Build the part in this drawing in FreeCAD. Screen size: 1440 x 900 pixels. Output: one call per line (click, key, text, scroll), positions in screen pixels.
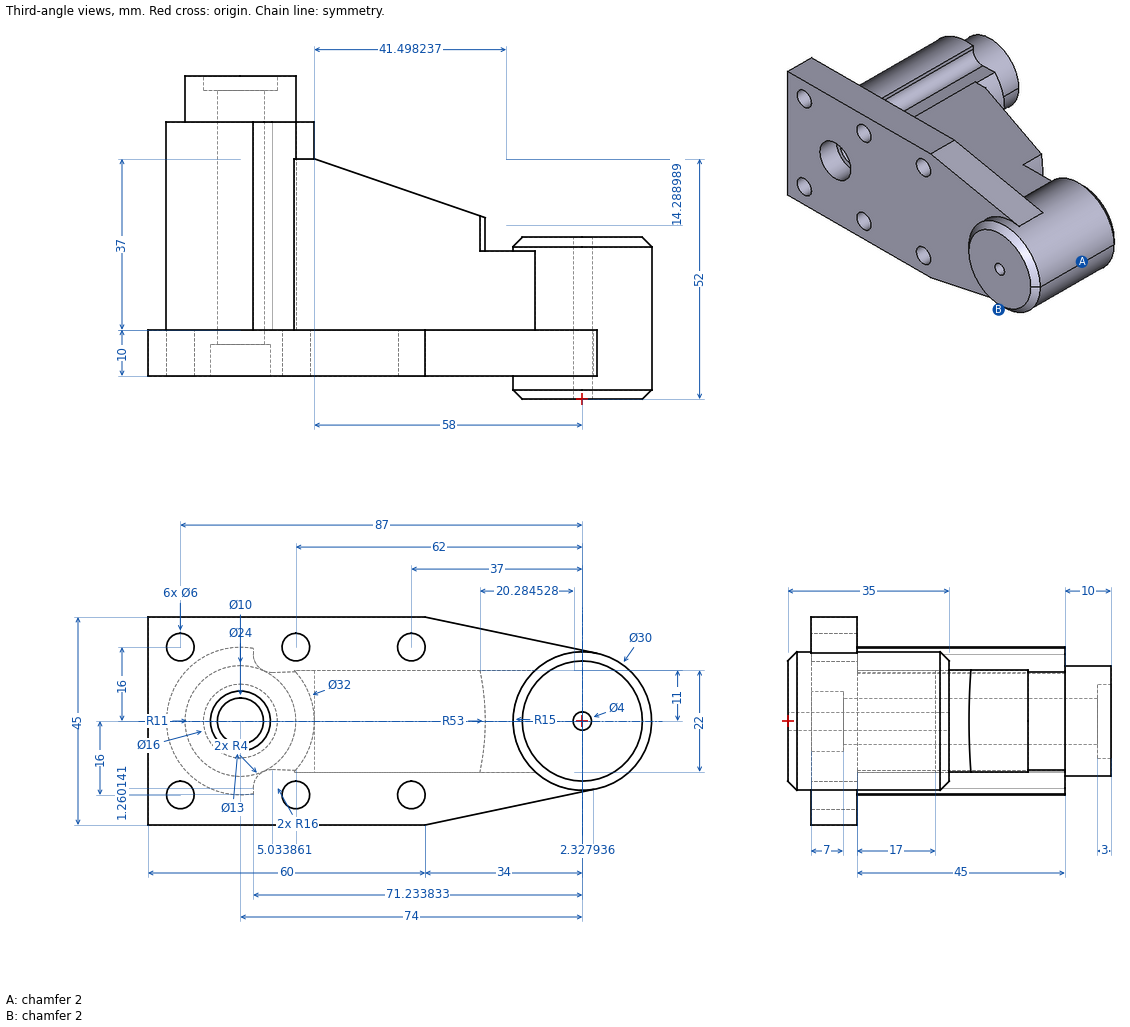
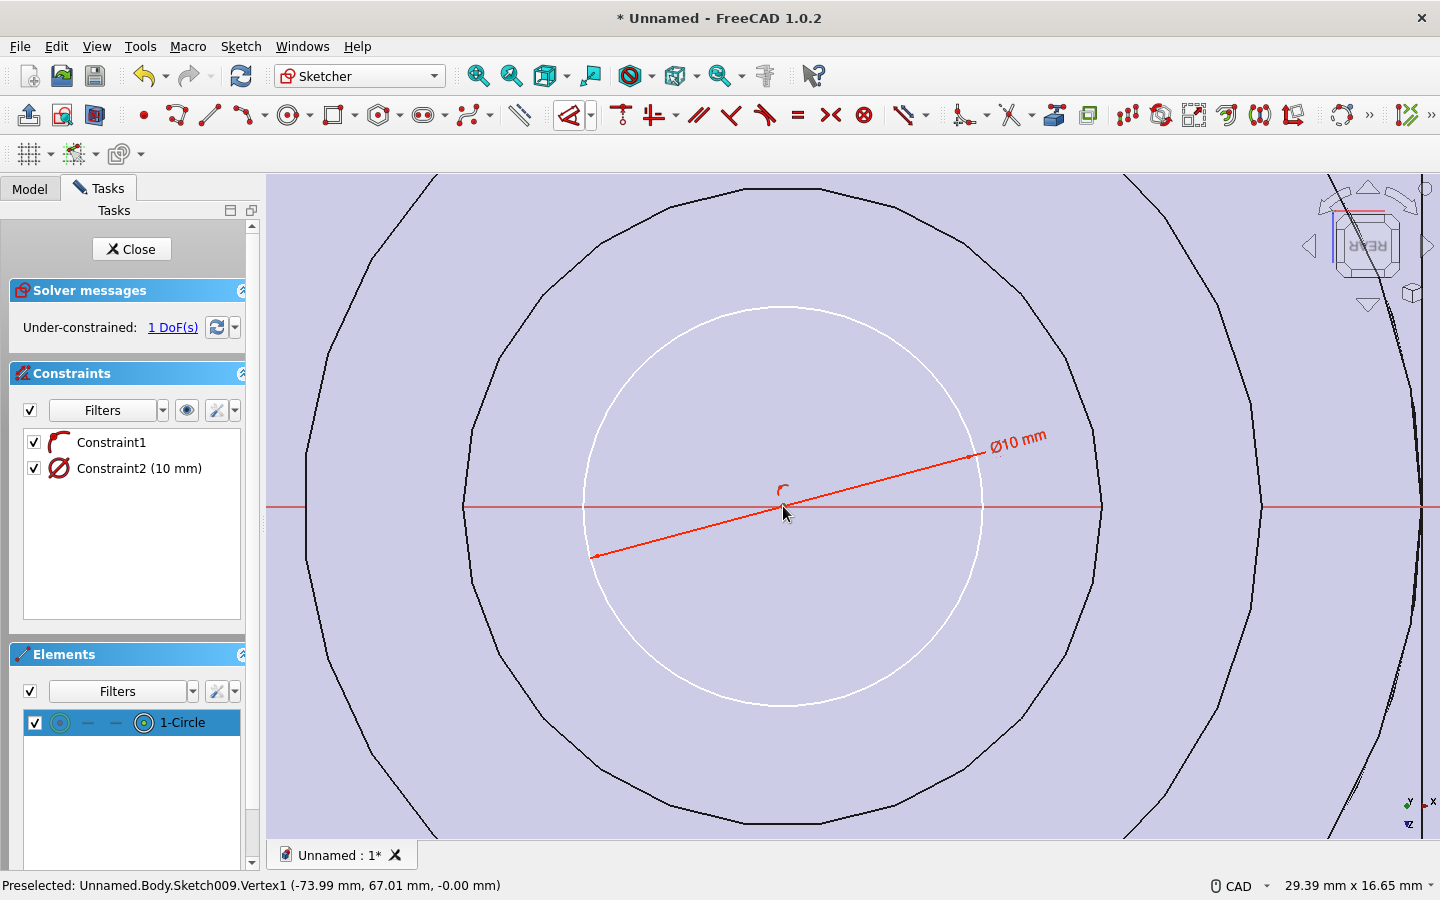
click(590, 116)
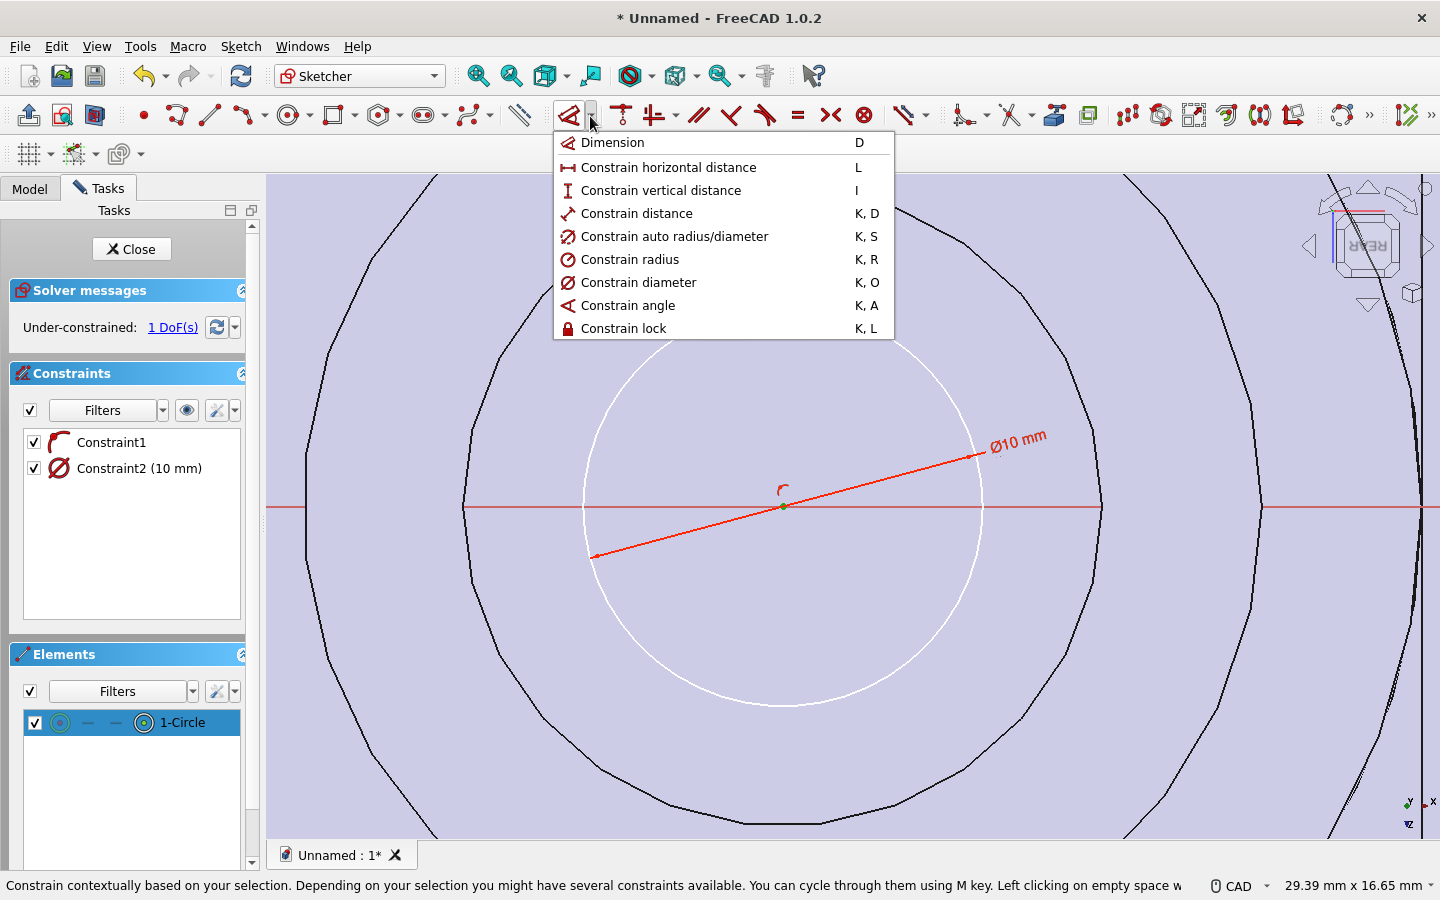
click(724, 168)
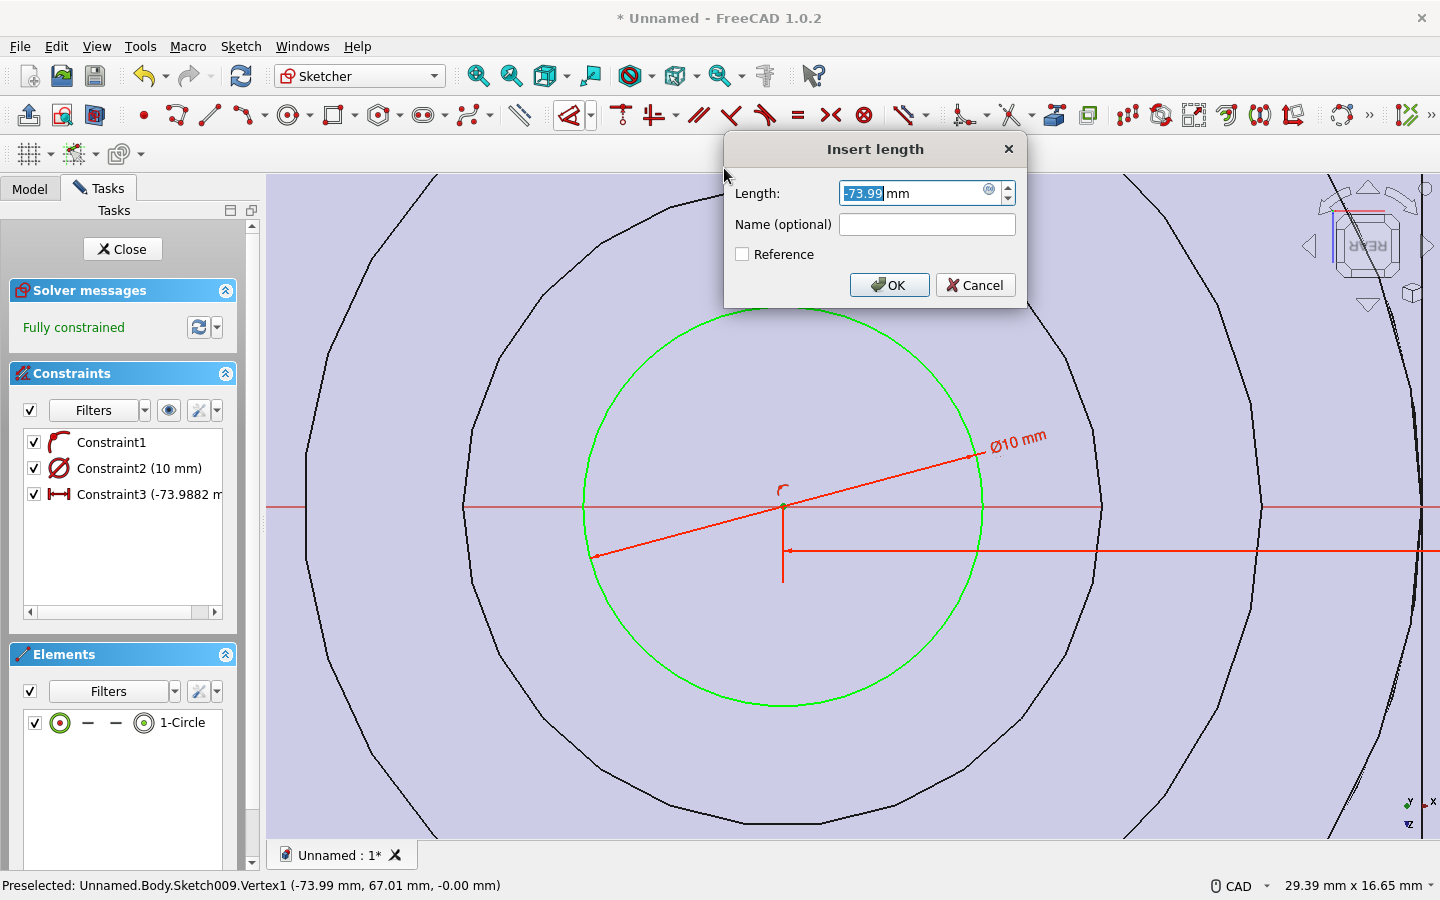
text(-74)
key(Return)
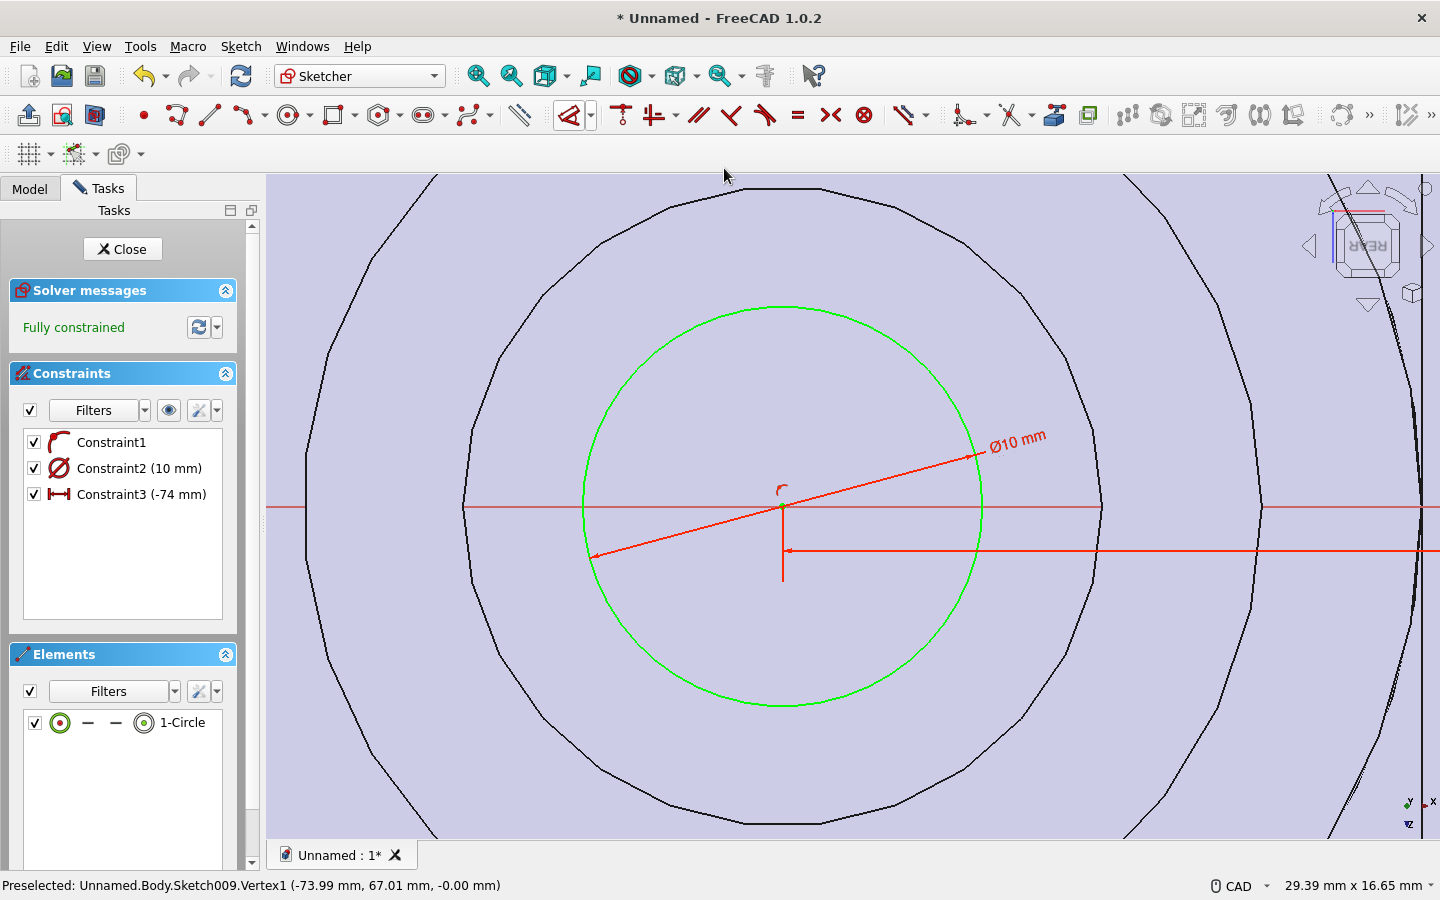
click(123, 249)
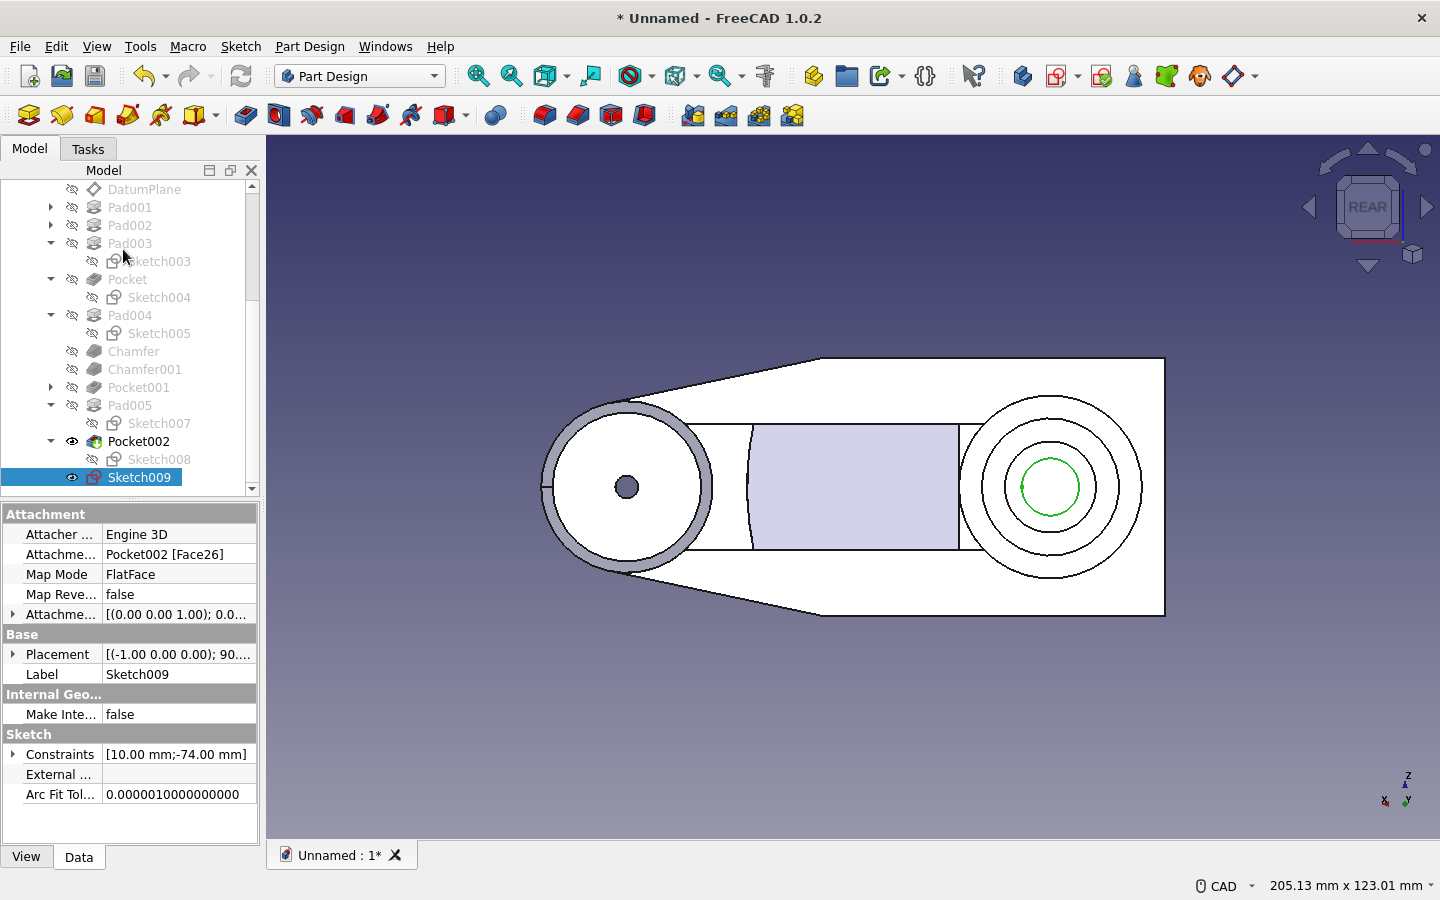
click(246, 116)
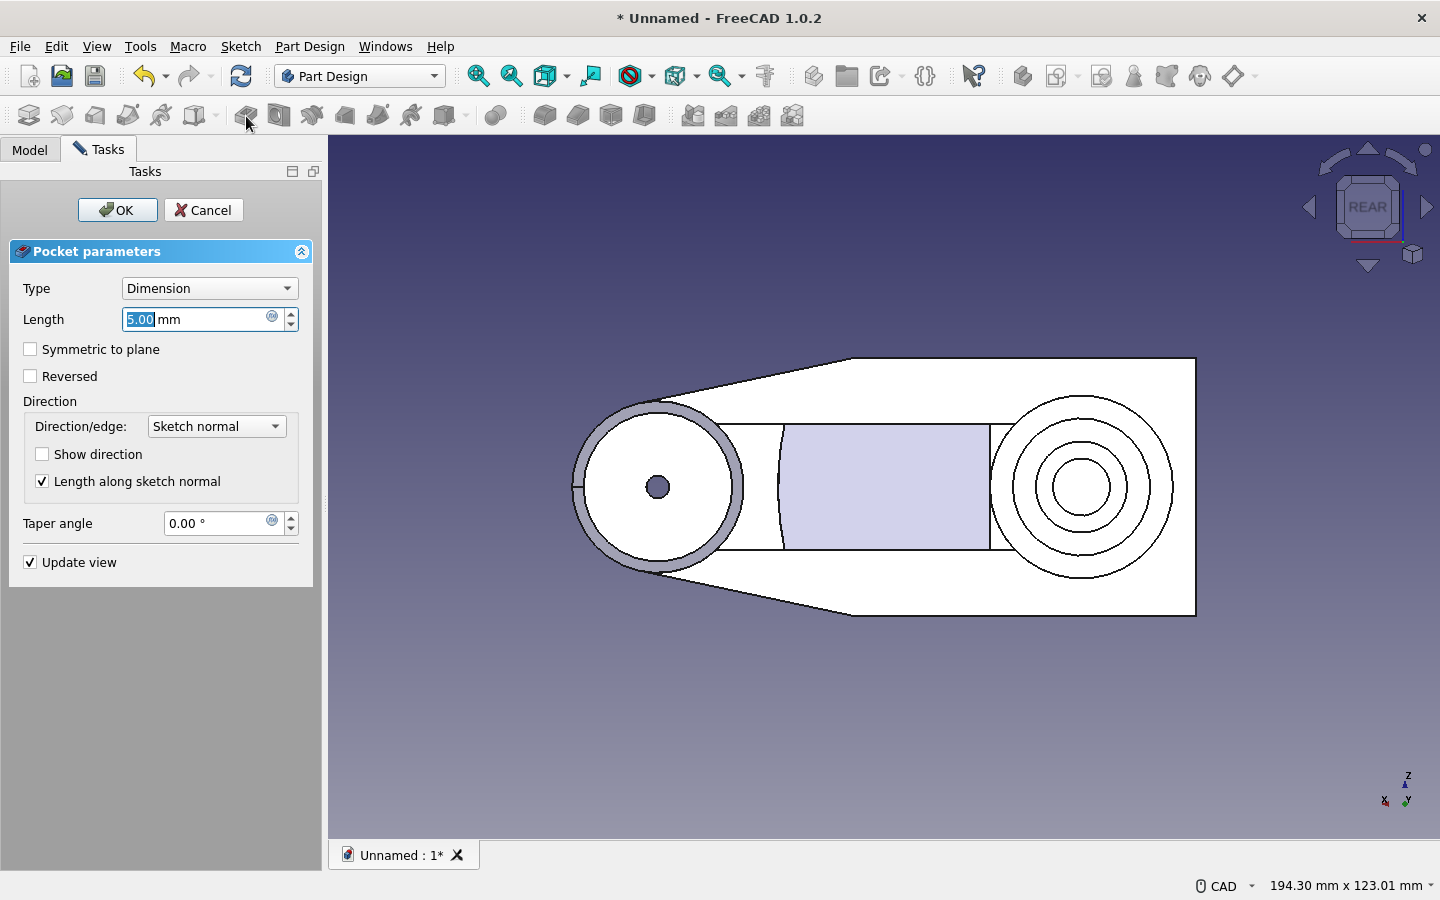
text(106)
key(Tab)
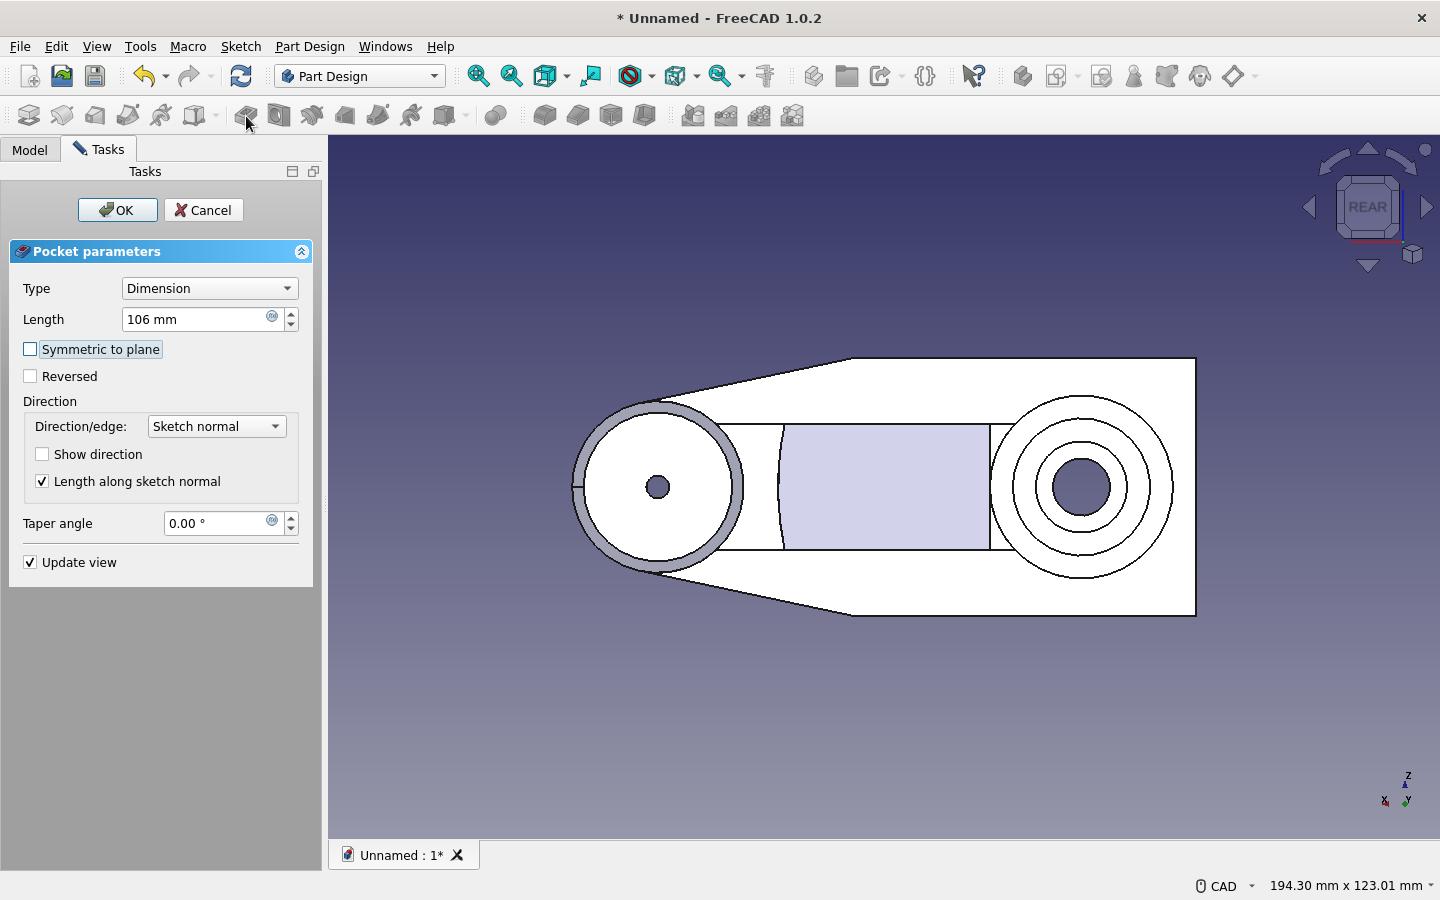
click(118, 210)